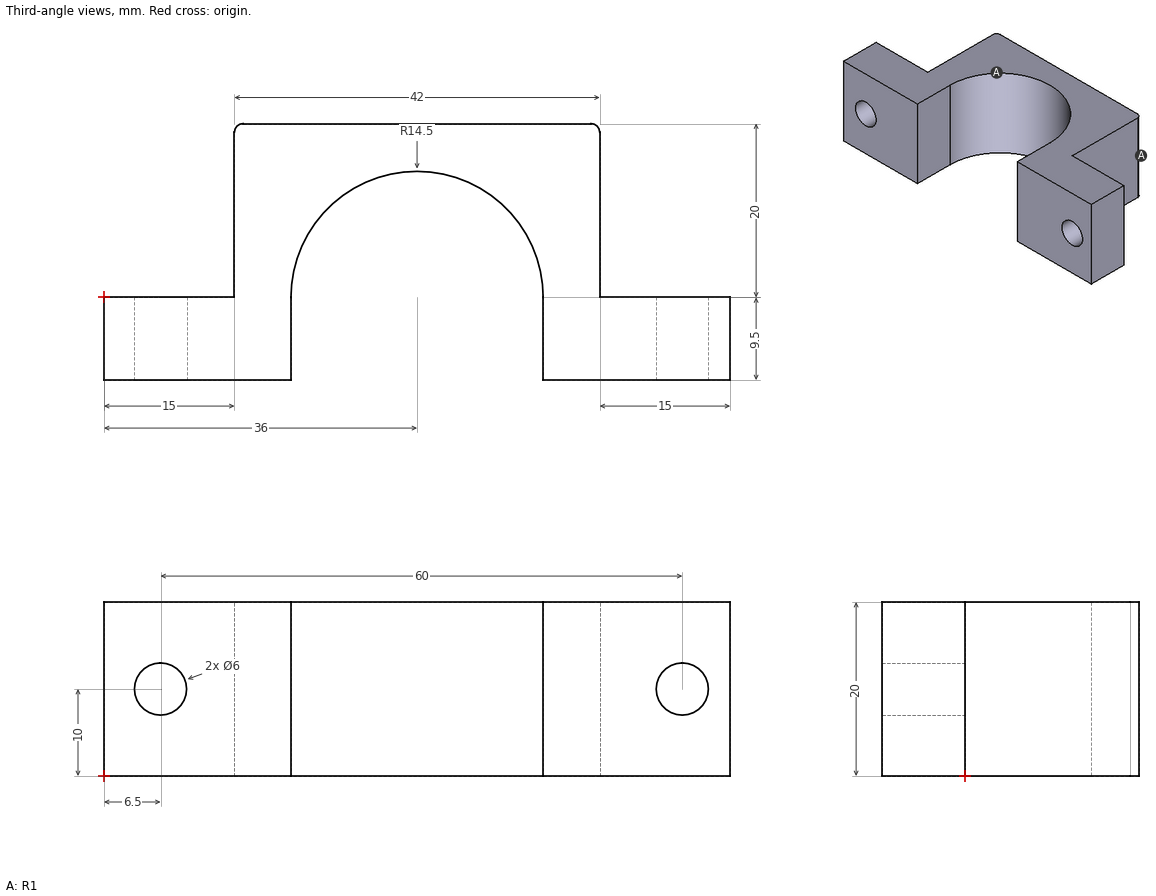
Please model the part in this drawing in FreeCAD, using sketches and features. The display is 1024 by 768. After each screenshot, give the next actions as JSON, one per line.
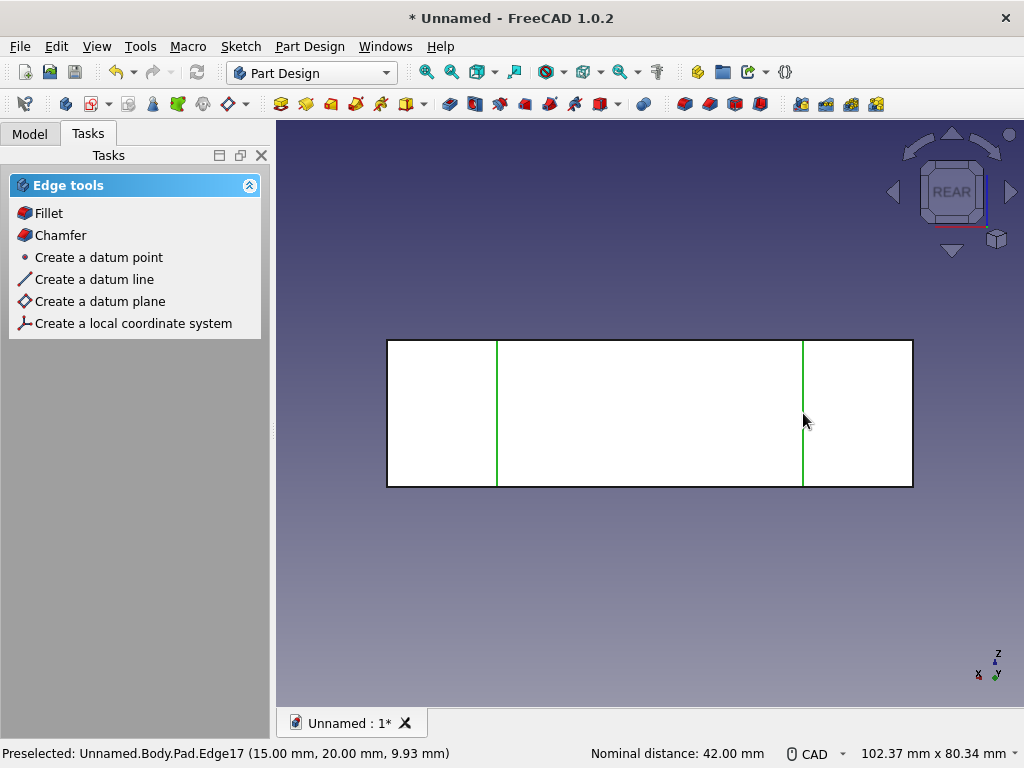
{"action": "left_click", "coordinate": [685, 104]}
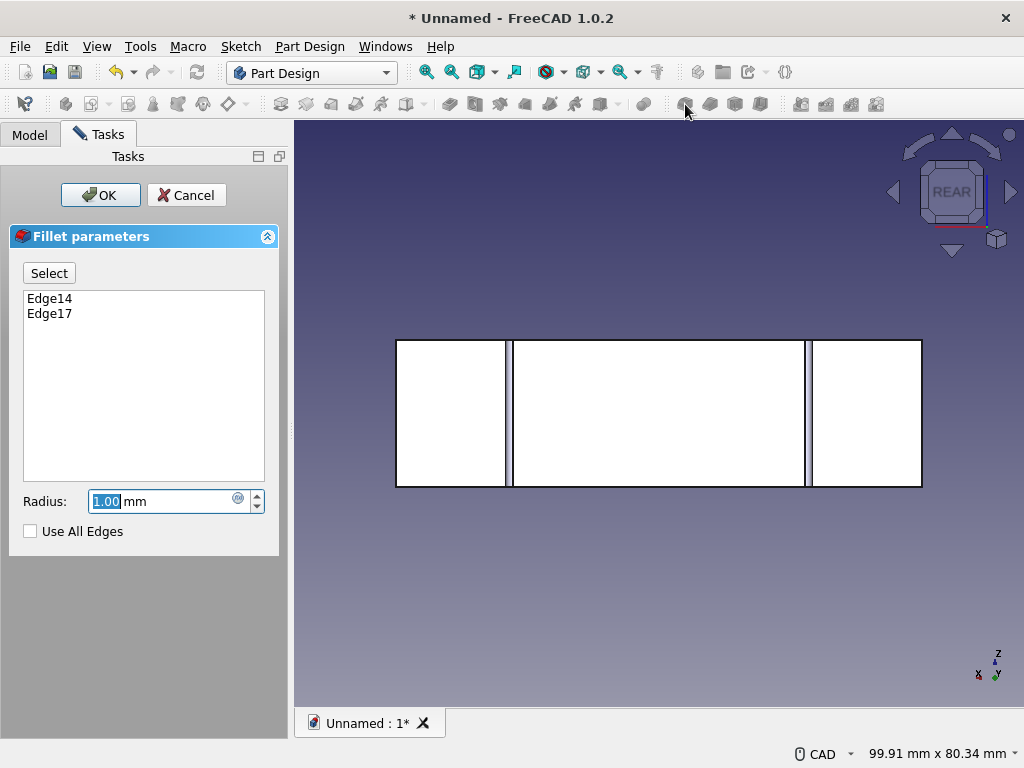
{"action": "type", "text": "1"}
{"action": "key", "text": "Tab"}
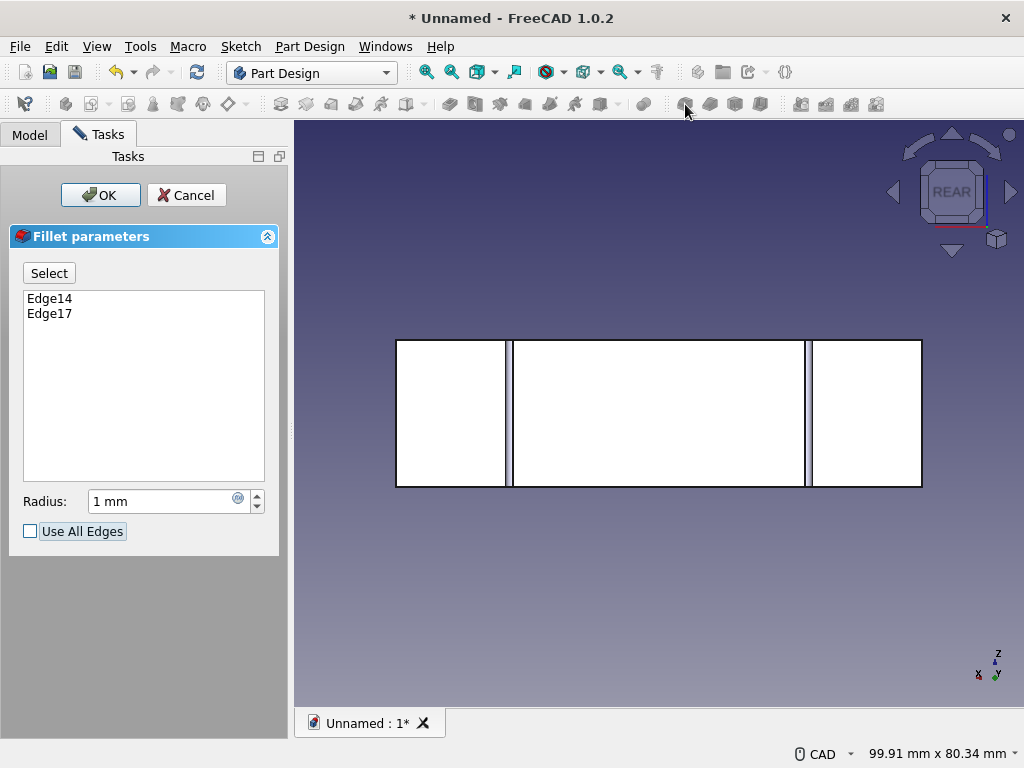
{"action": "left_click", "coordinate": [101, 195]}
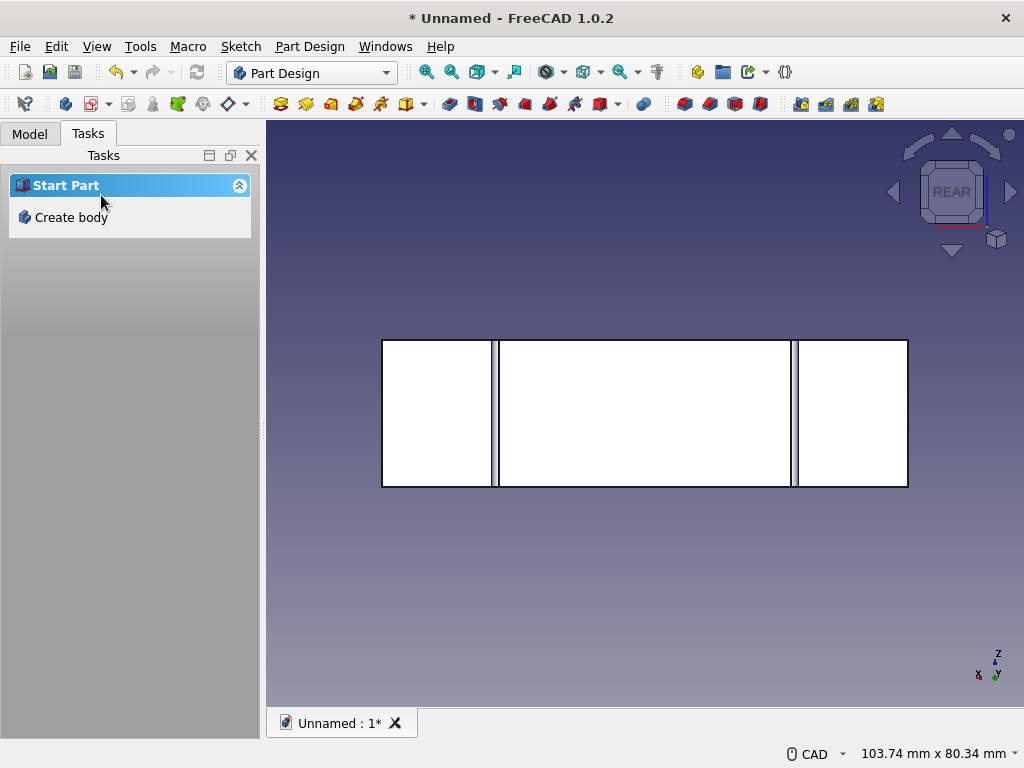
{"action": "left_click", "coordinate": [90, 104]}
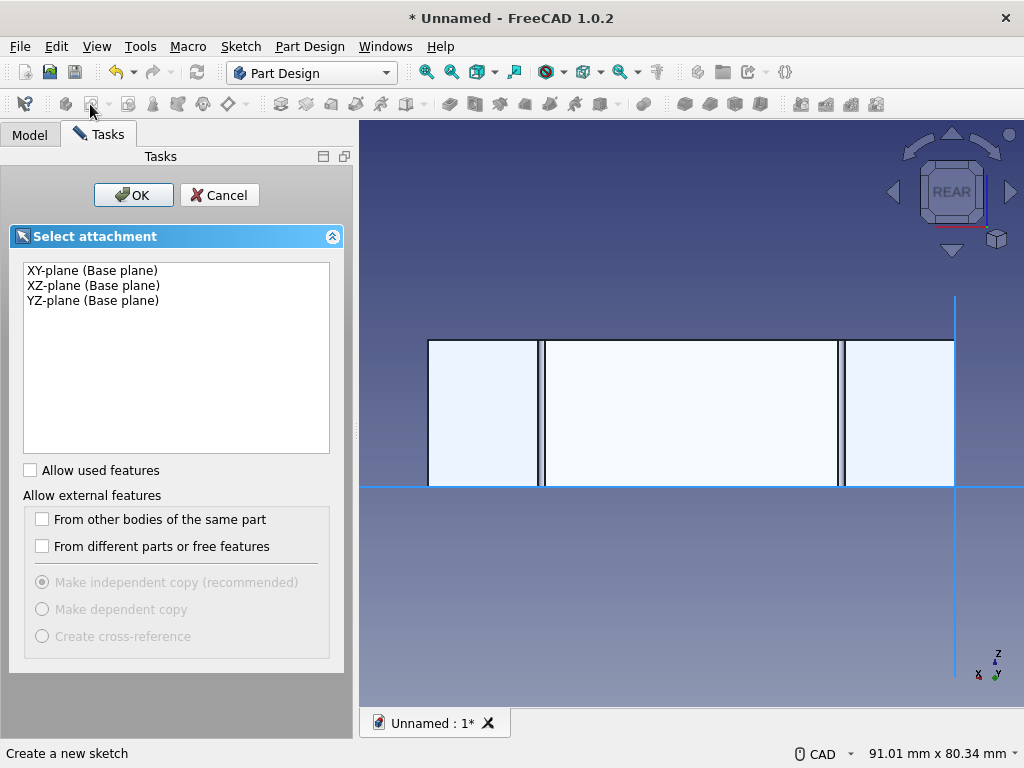
{"action": "left_click", "coordinate": [84, 286]}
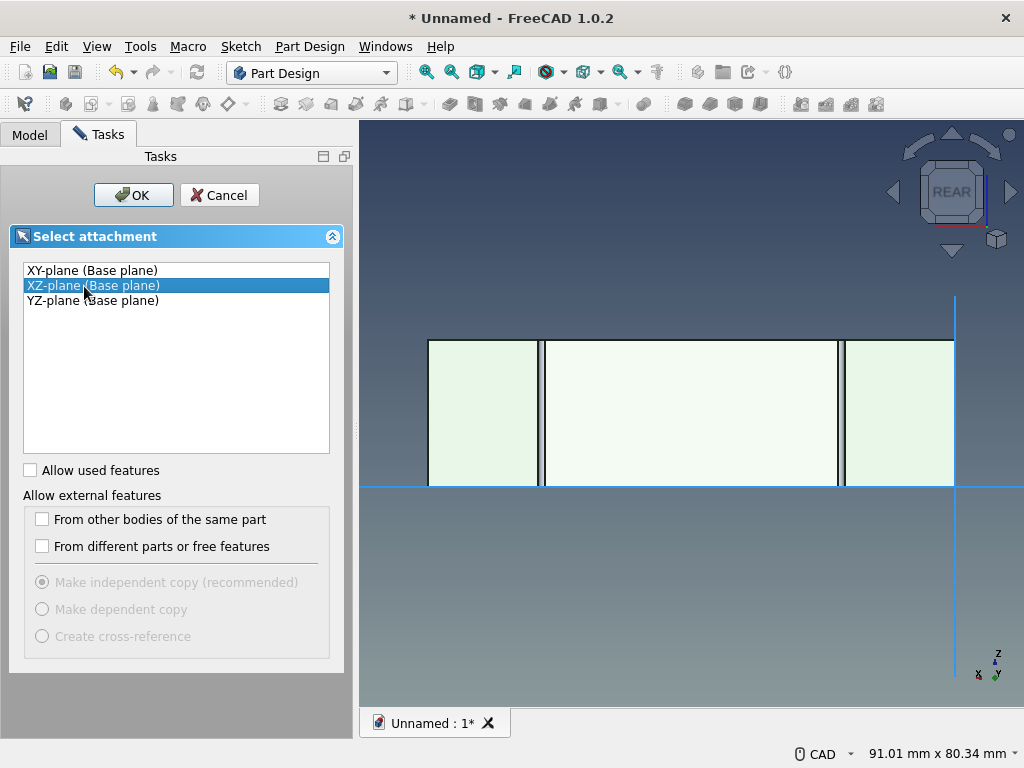
{"action": "left_click", "coordinate": [134, 195]}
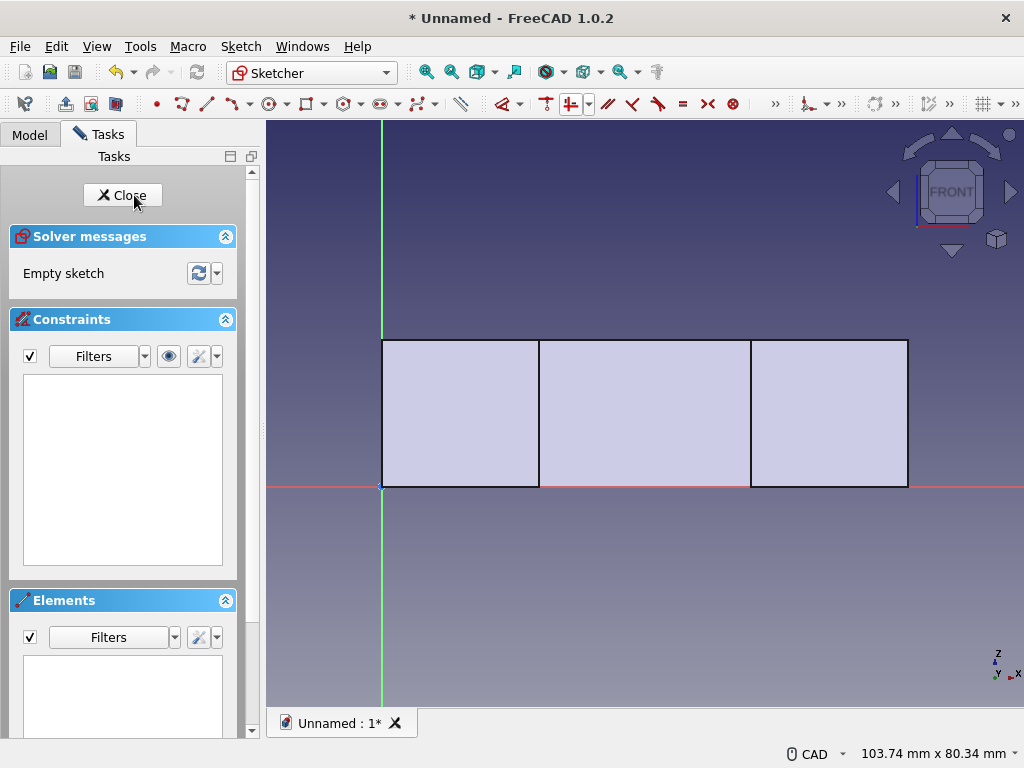
{"action": "left_click", "coordinate": [116, 104]}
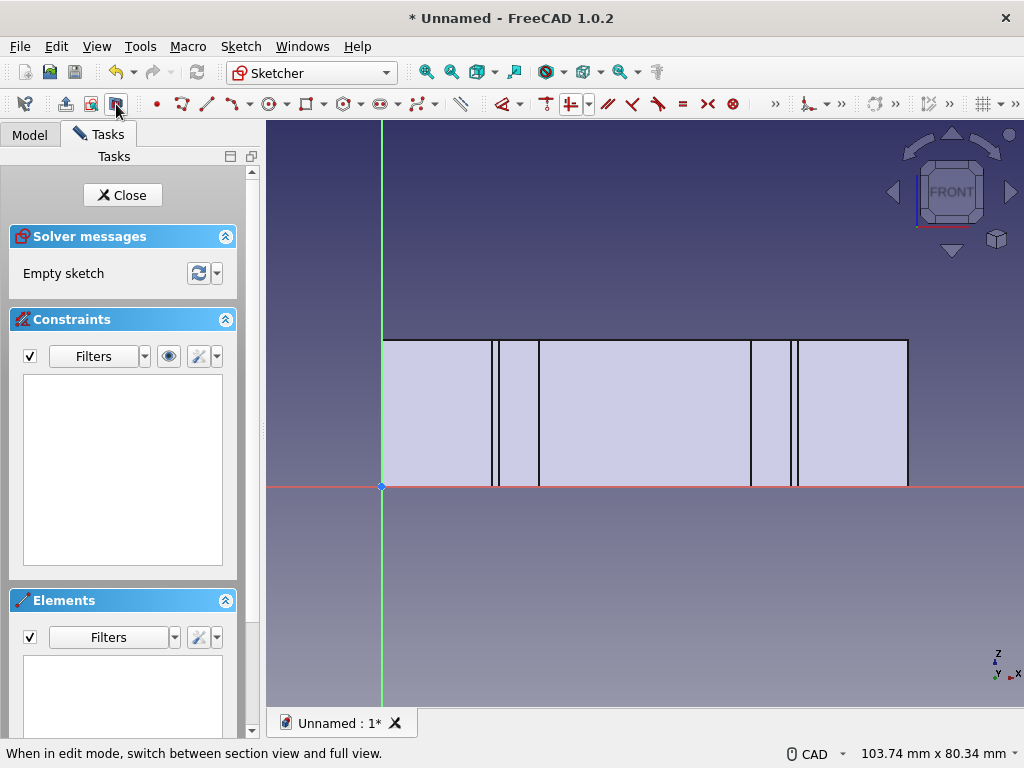
{"action": "scroll", "coordinate": [308, 298], "scroll_direction": "down", "scroll_amount": 1}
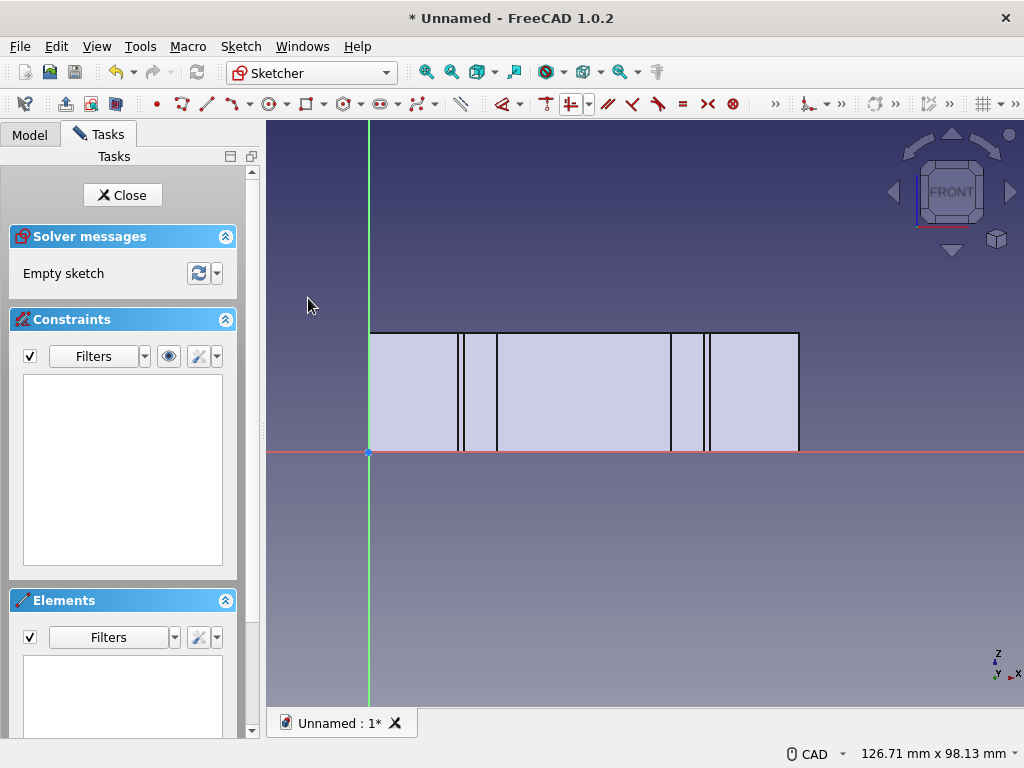
{"action": "left_click", "coordinate": [268, 104]}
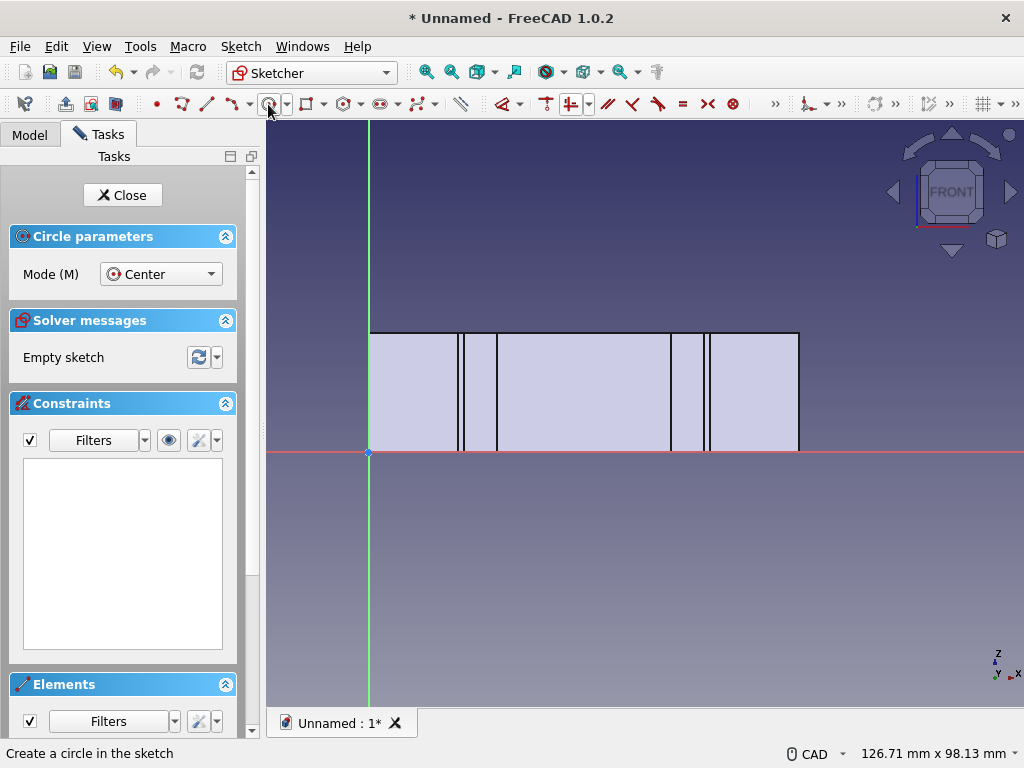
{"action": "scroll", "coordinate": [407, 393], "scroll_direction": "up", "scroll_amount": 2}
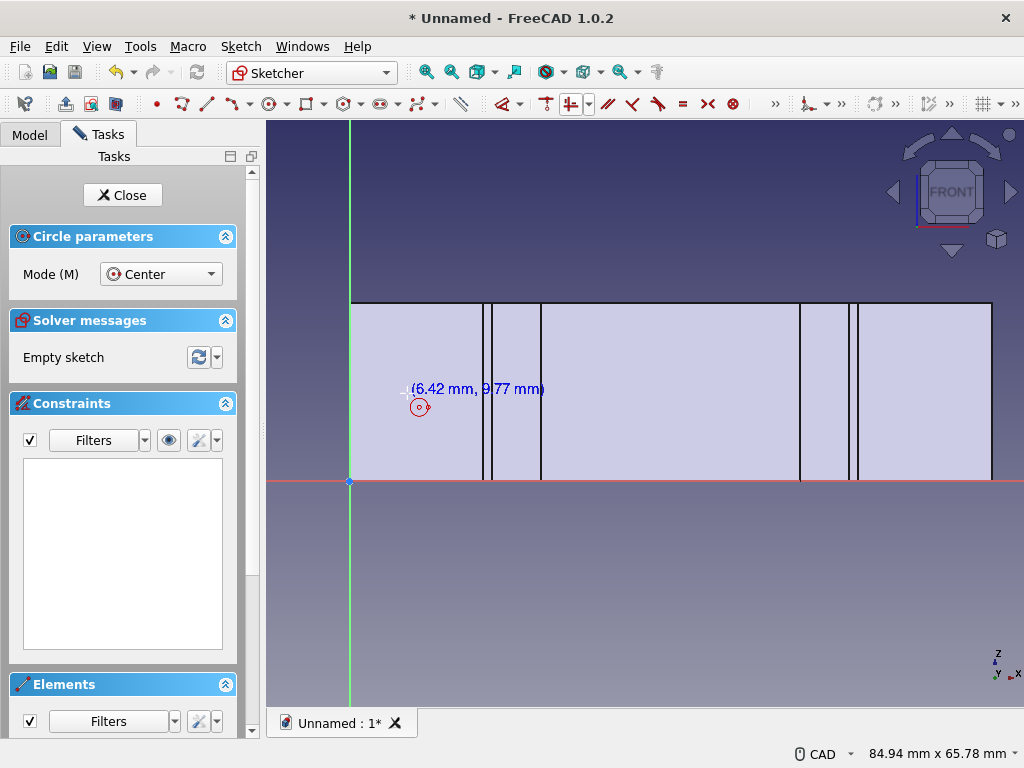
{"action": "left_click", "coordinate": [408, 392]}
{"action": "left_click", "coordinate": [427, 373]}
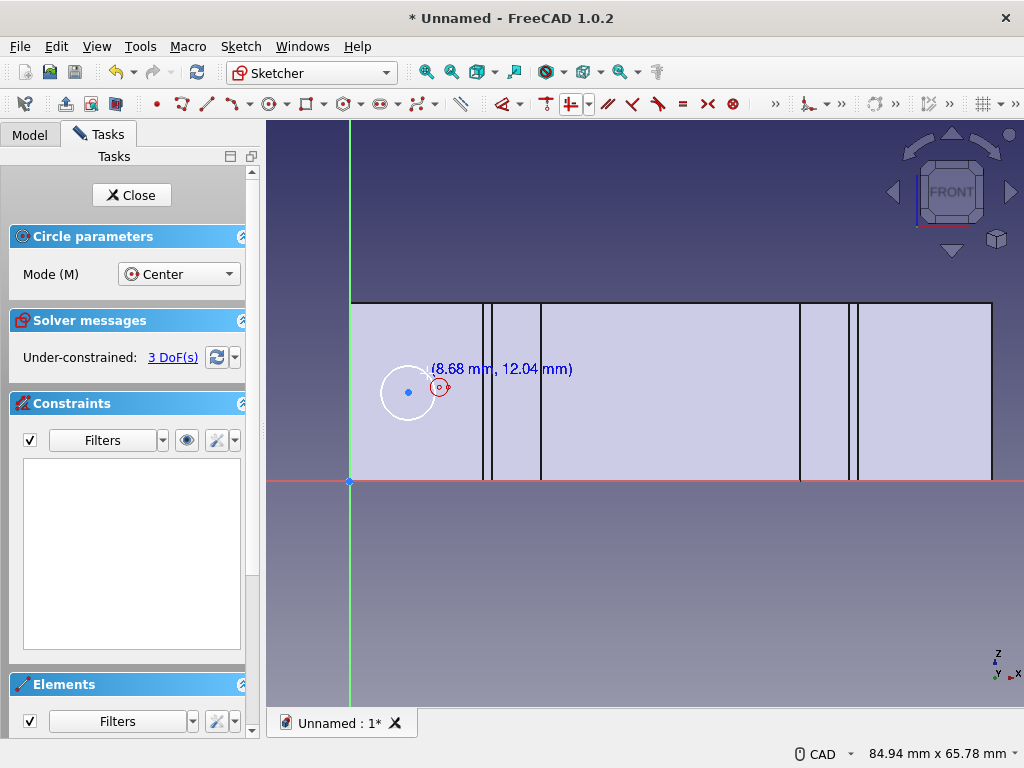
{"action": "scroll", "coordinate": [407, 393], "scroll_direction": "down", "scroll_amount": 2}